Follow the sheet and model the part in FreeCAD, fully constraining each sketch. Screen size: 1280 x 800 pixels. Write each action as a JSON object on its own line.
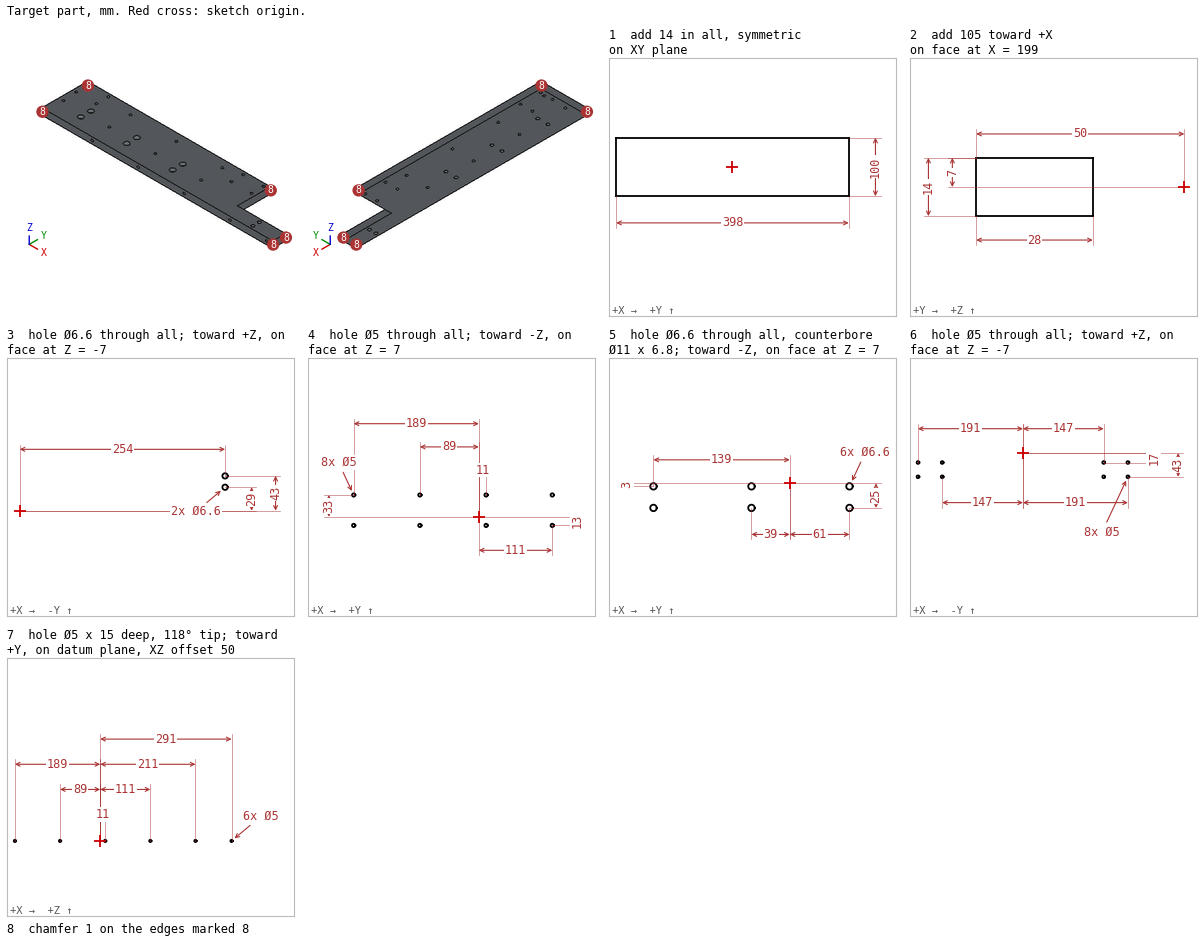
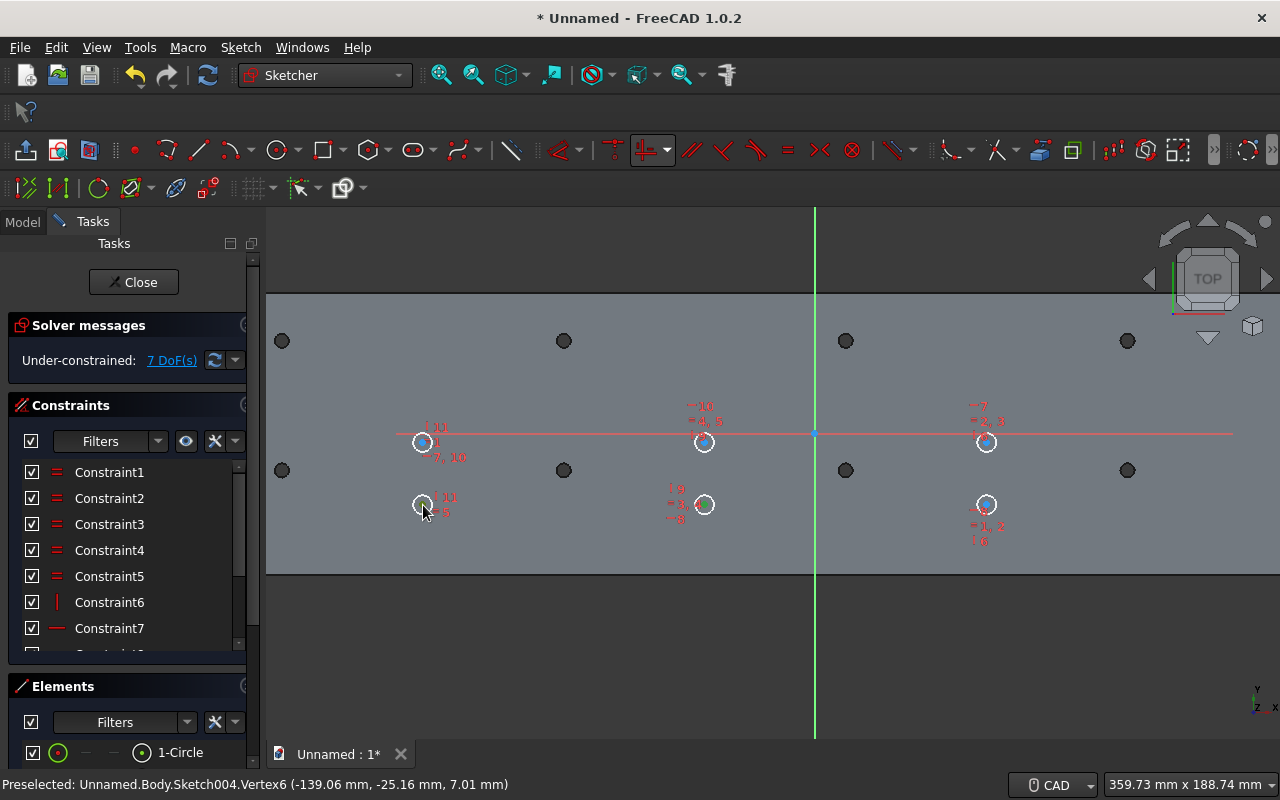
{"action": "left_click", "coordinate": [670, 150]}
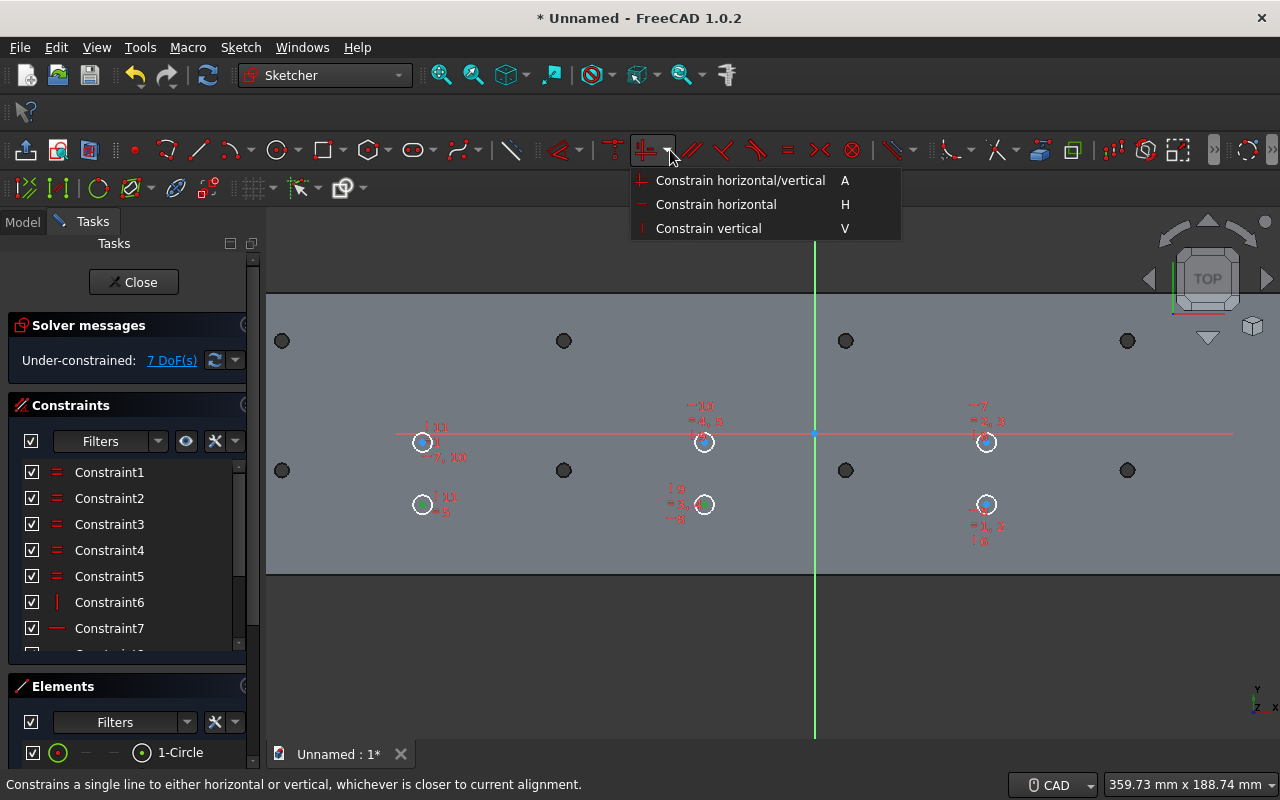
{"action": "left_click", "coordinate": [766, 204]}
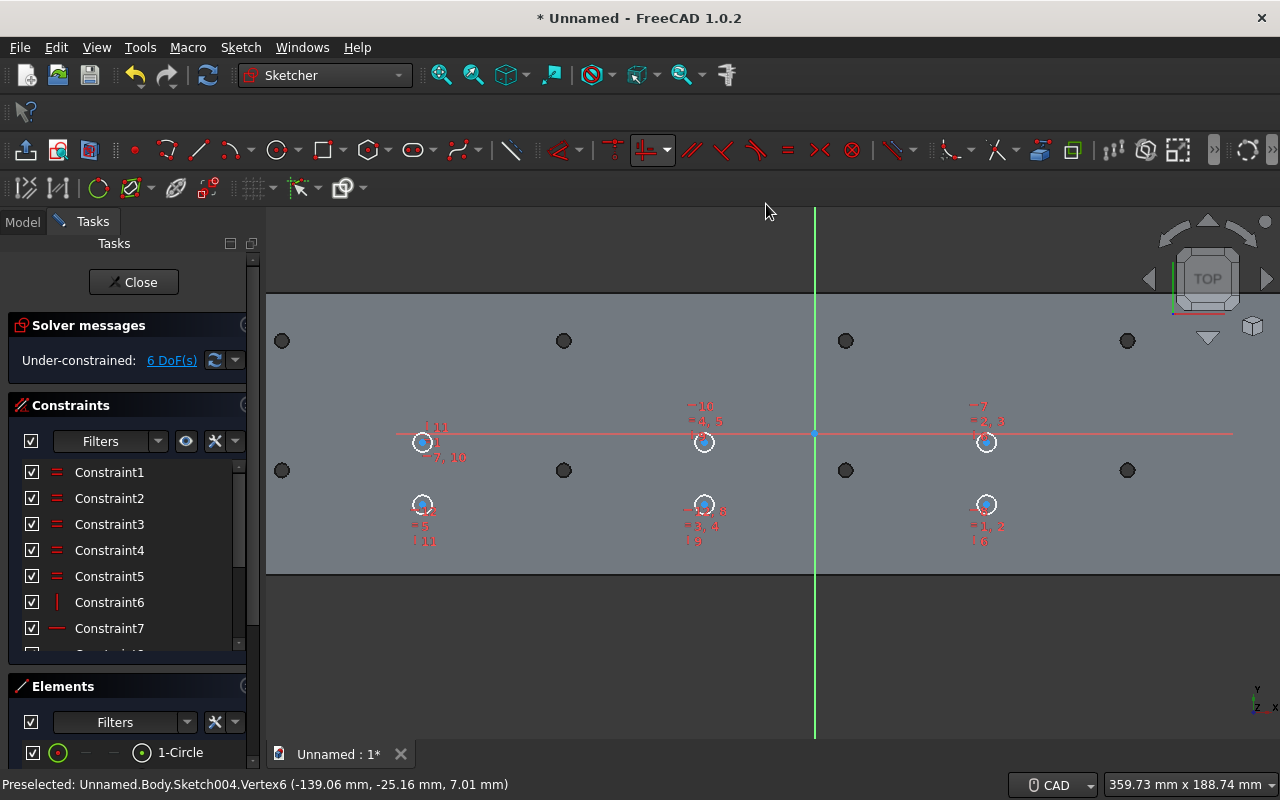
{"action": "key", "text": "d"}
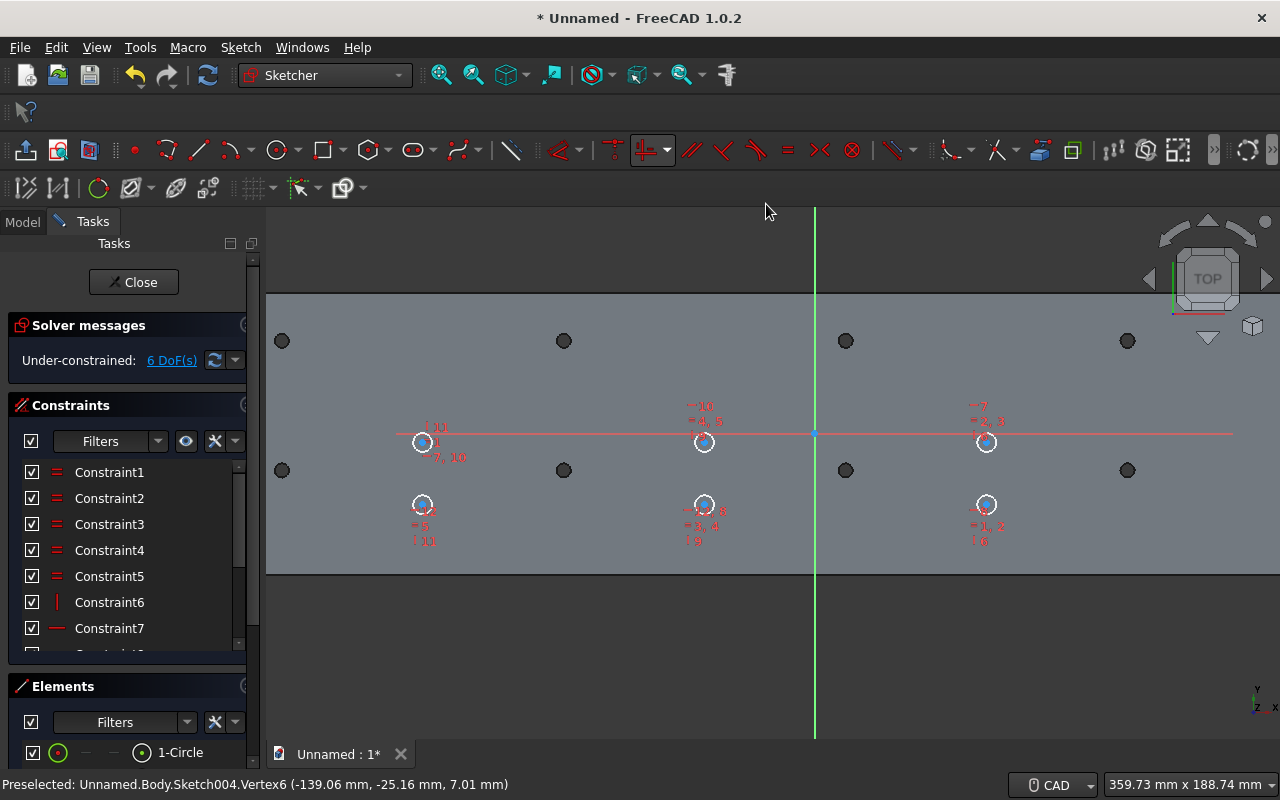
{"action": "scroll", "coordinate": [429, 436], "scroll_direction": "up", "scroll_amount": 4}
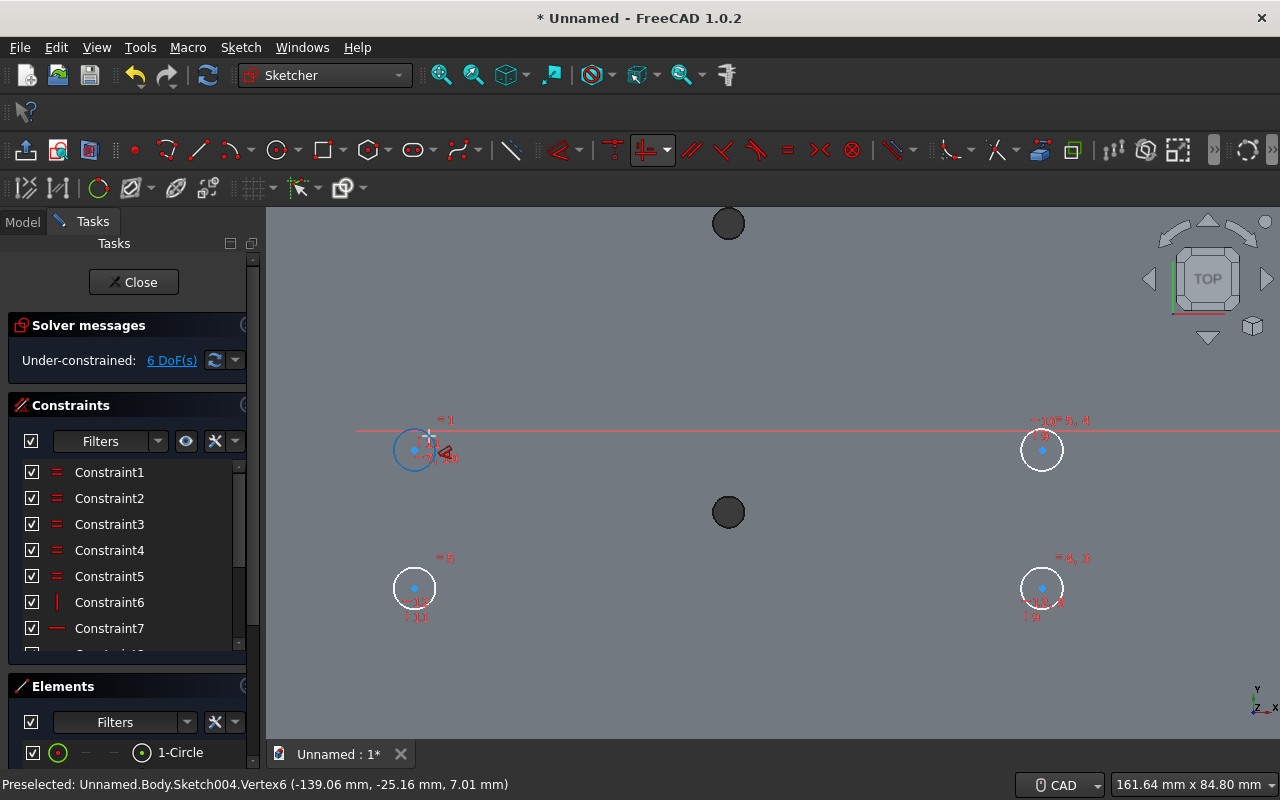
{"action": "left_click", "coordinate": [429, 435]}
{"action": "left_click", "coordinate": [451, 412]}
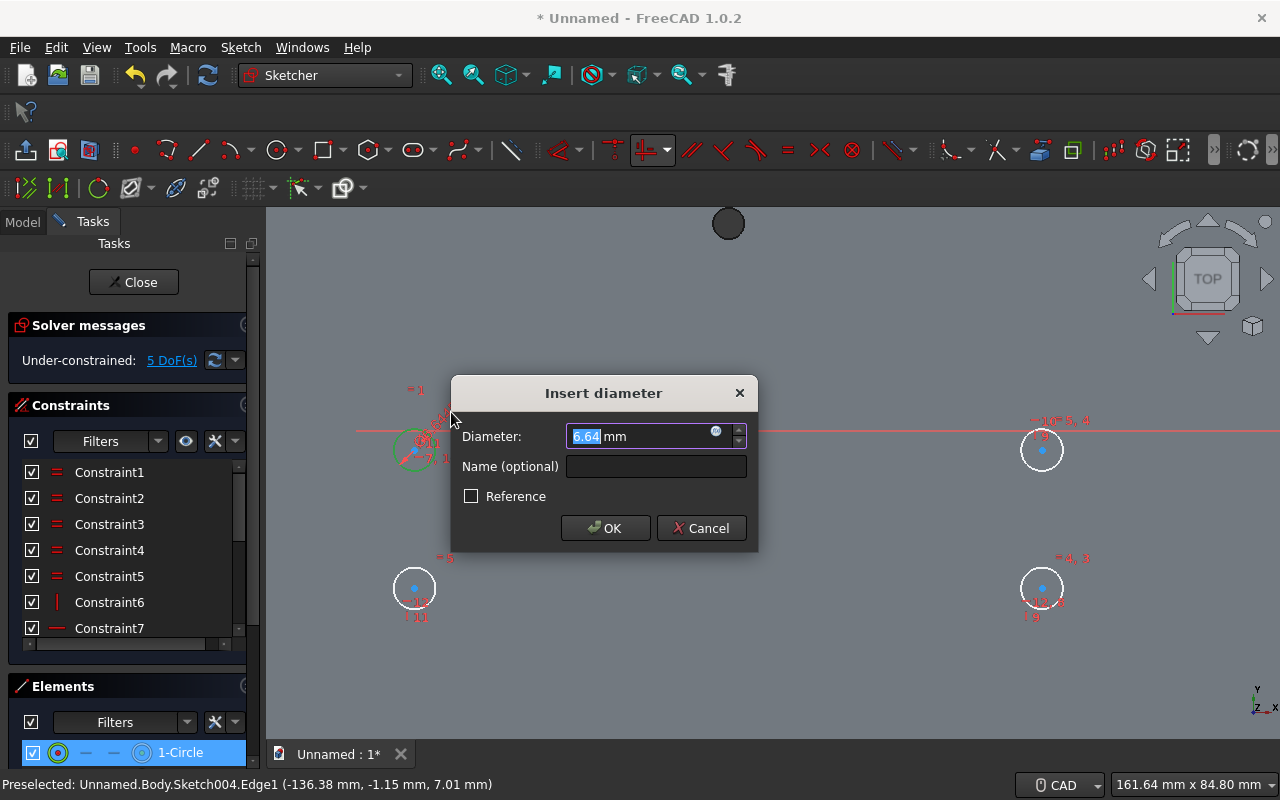
{"action": "type", "text": "6.6"}
{"action": "key", "text": "Return"}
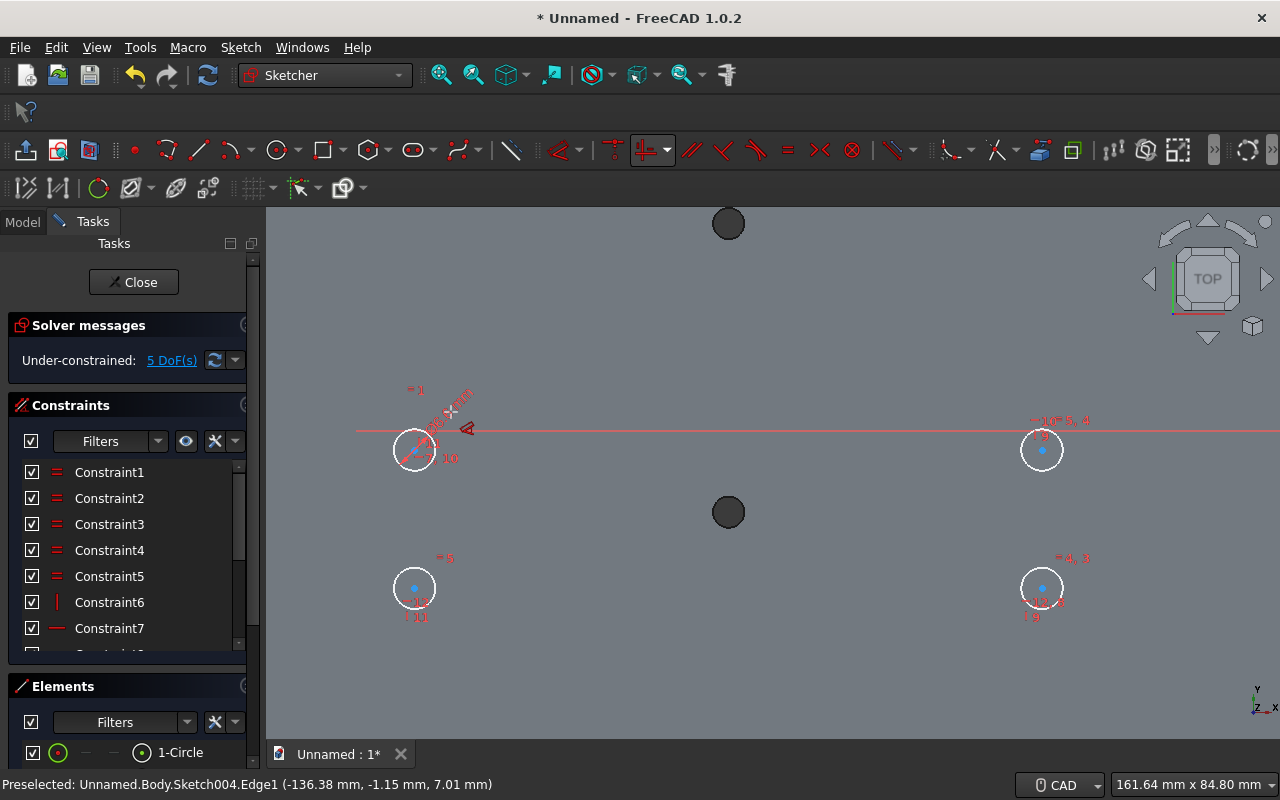
{"action": "scroll", "coordinate": [415, 450], "scroll_direction": "up", "scroll_amount": 4}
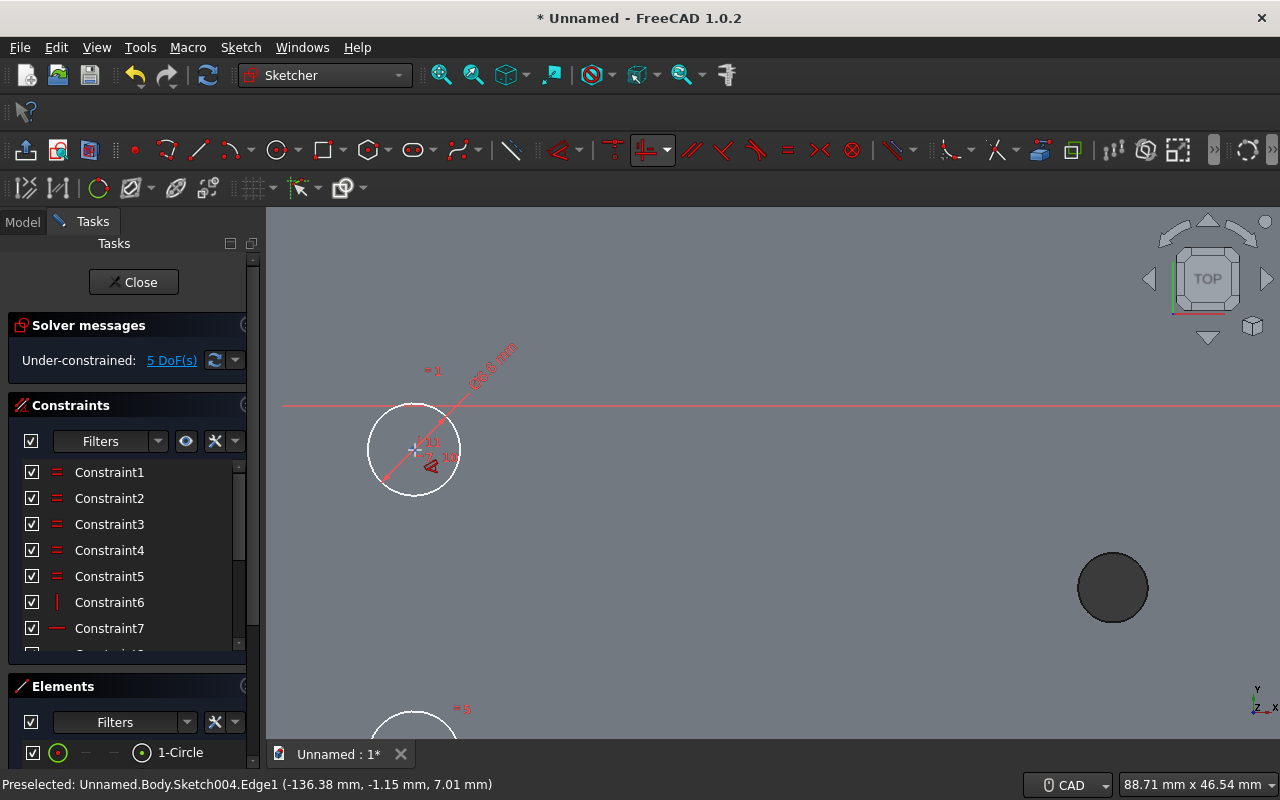
{"action": "left_click", "coordinate": [414, 450]}
{"action": "left_click", "coordinate": [356, 428]}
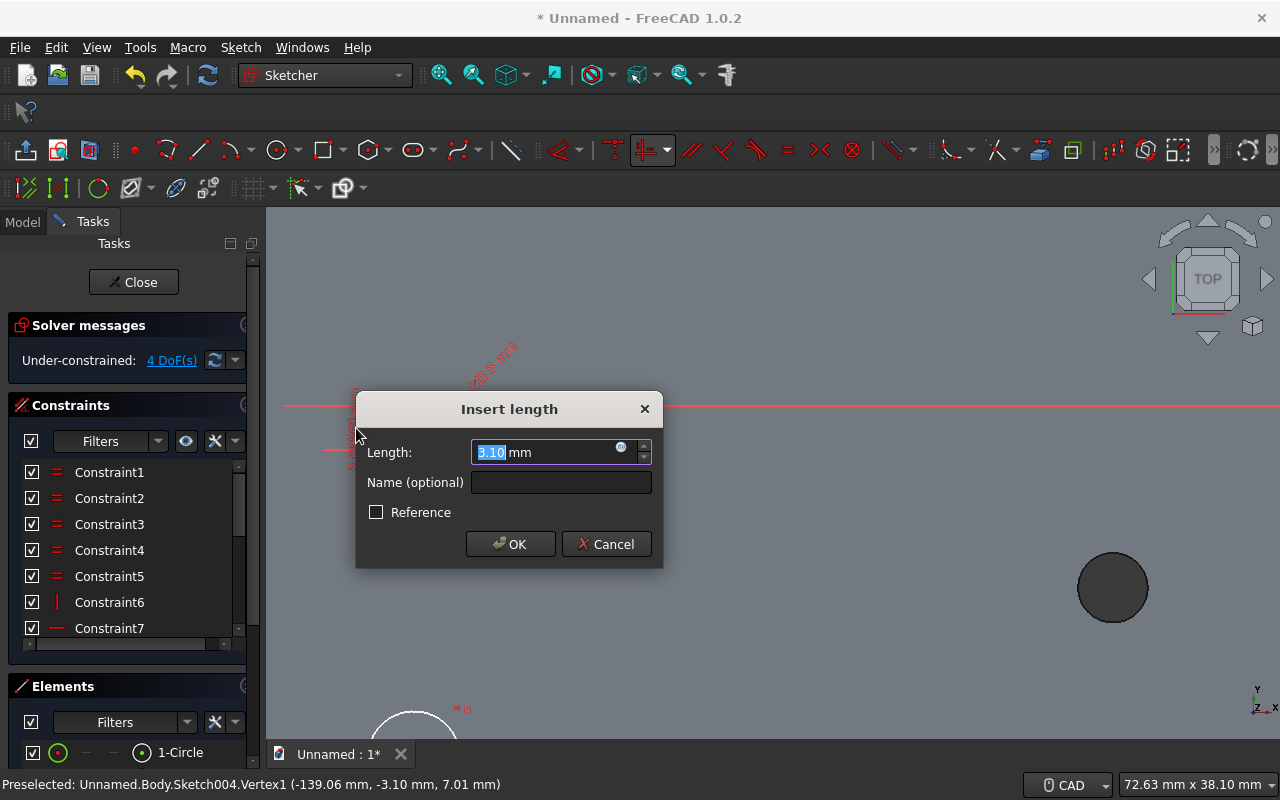
{"action": "type", "text": "3"}
{"action": "key", "text": "Return"}